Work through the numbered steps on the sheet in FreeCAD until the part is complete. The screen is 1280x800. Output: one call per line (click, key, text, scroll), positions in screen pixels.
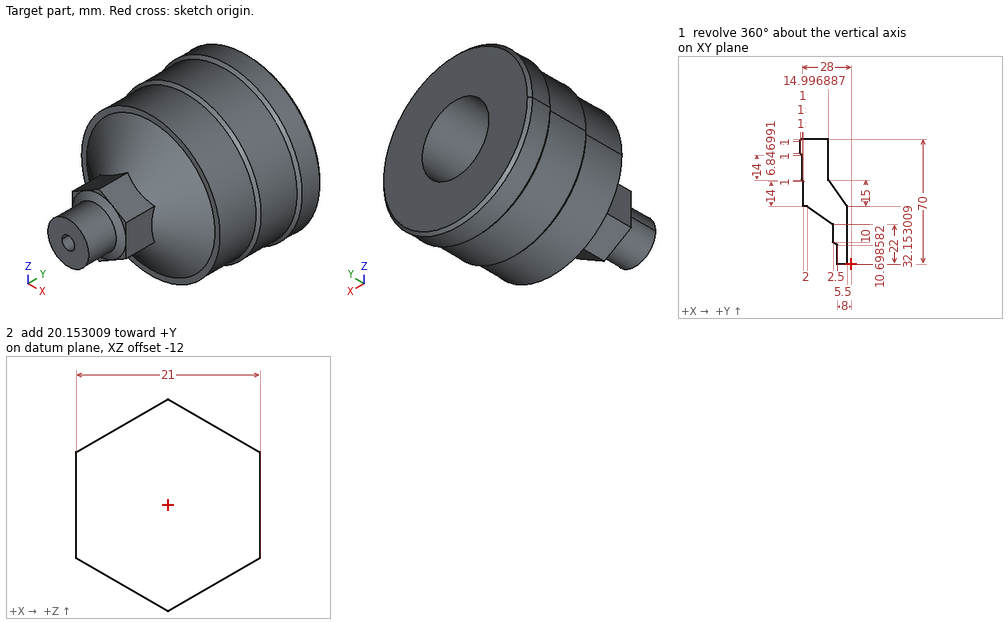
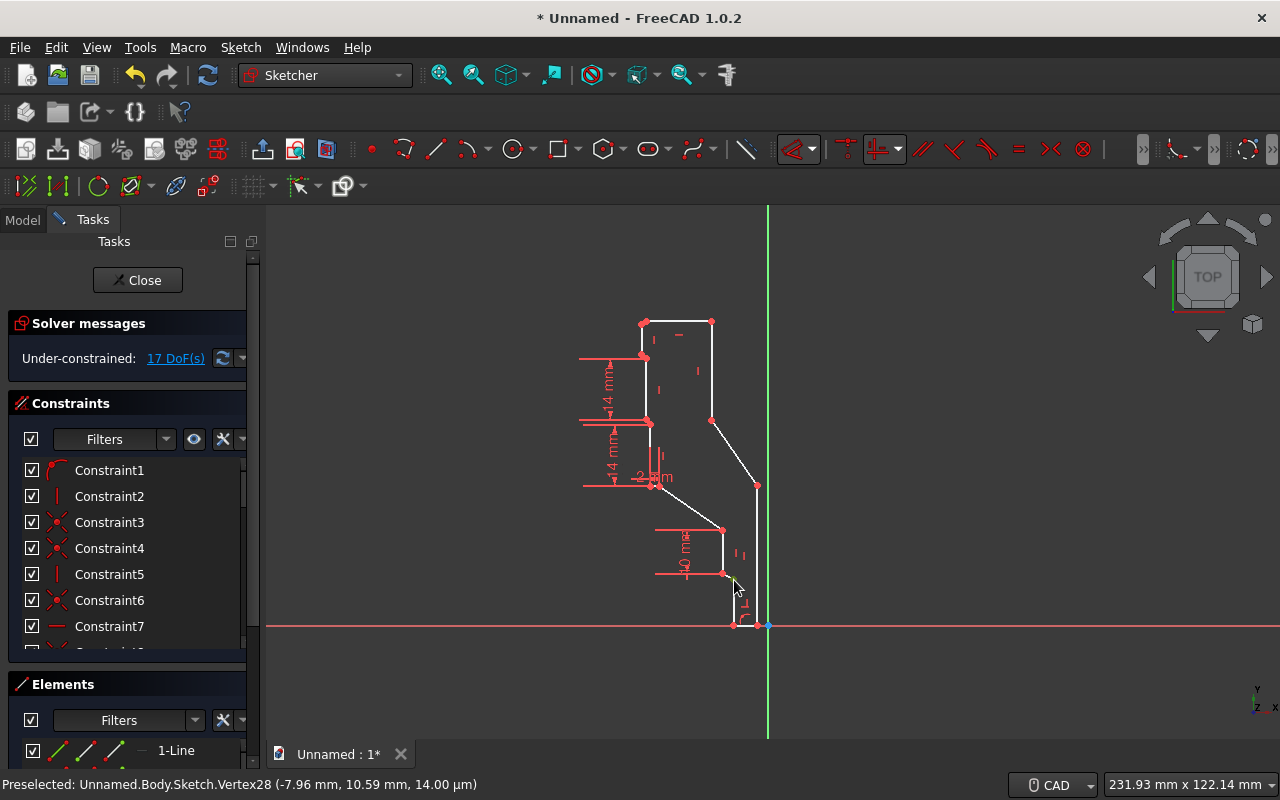
key(l)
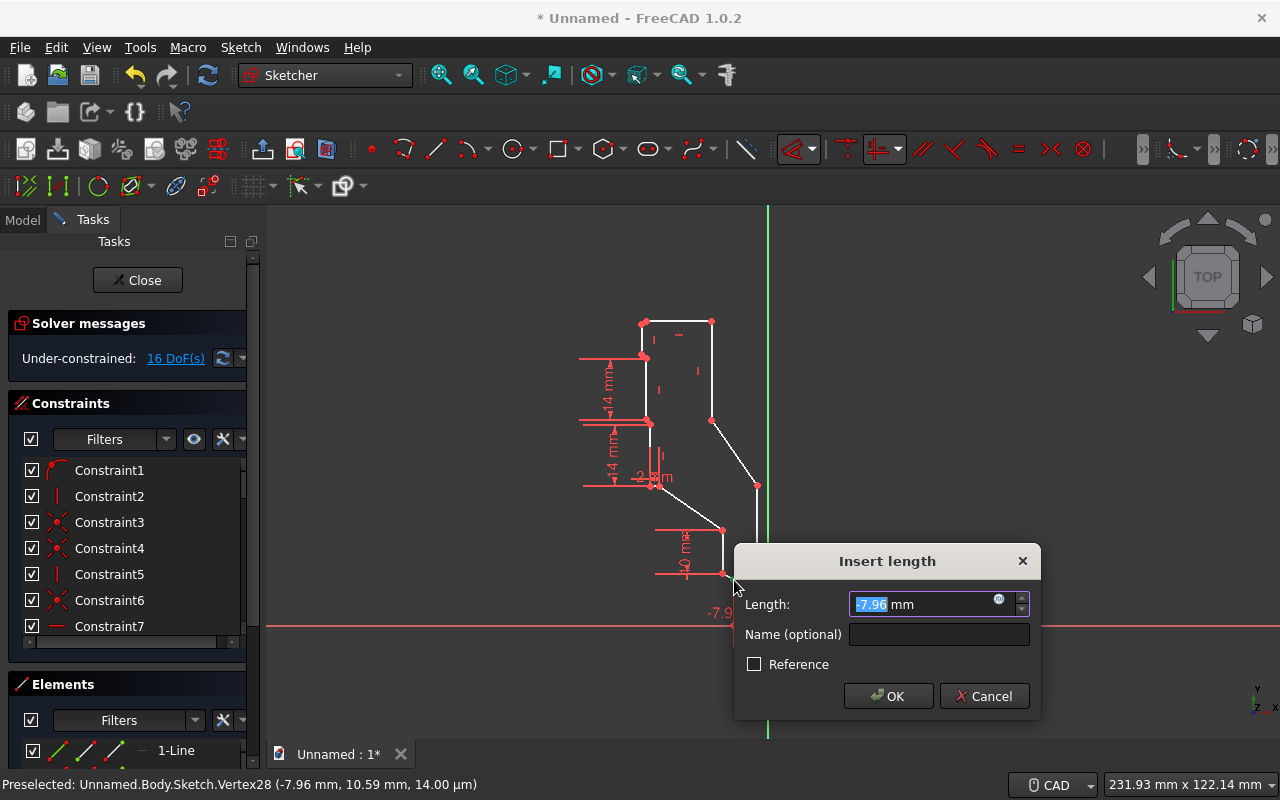
text(-8)
key(Return)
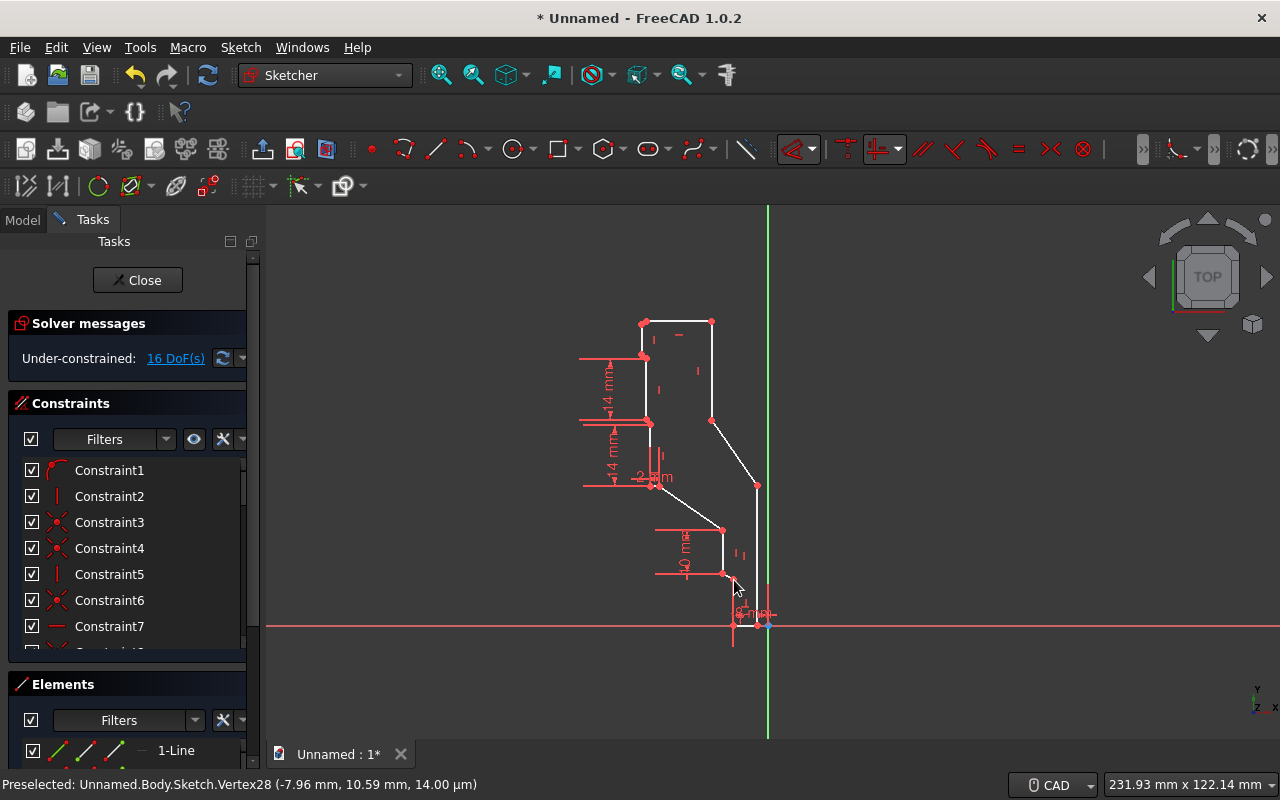
scroll(644, 323, up, 12)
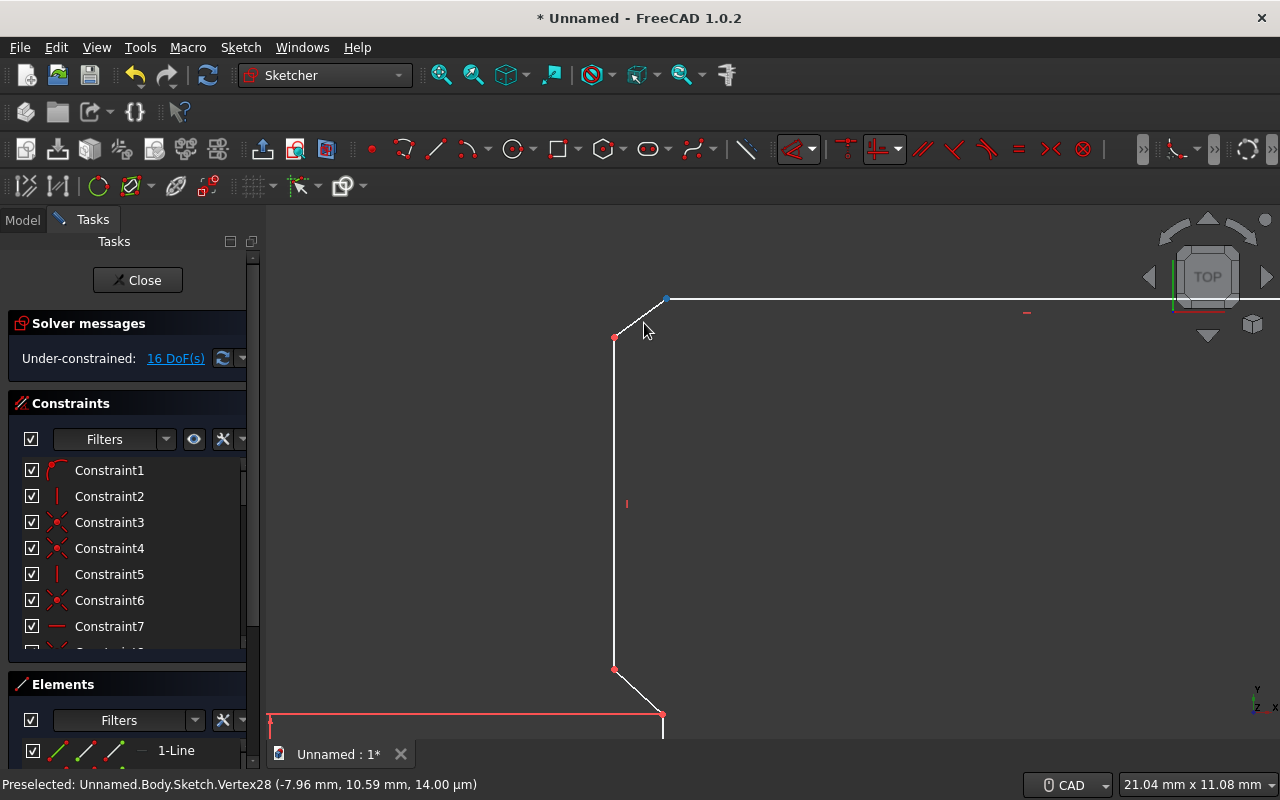
click(640, 318)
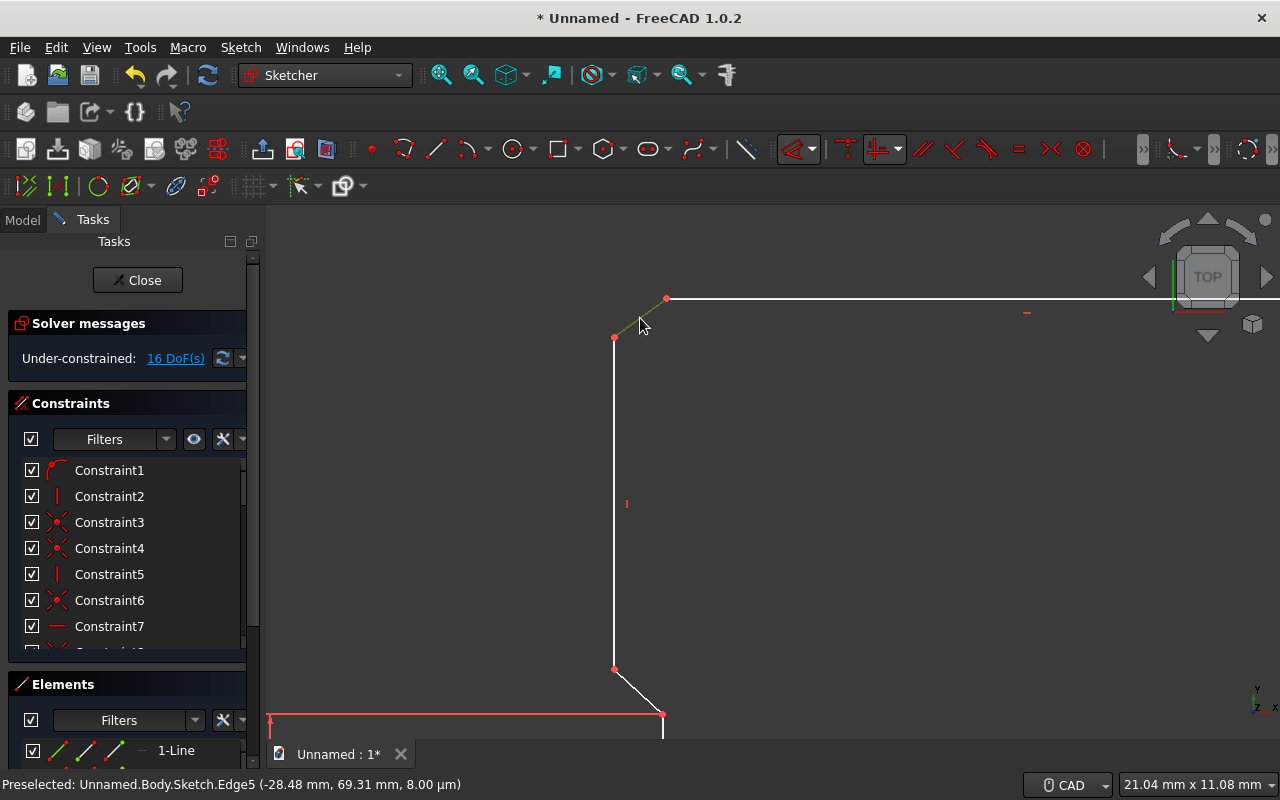
click(814, 150)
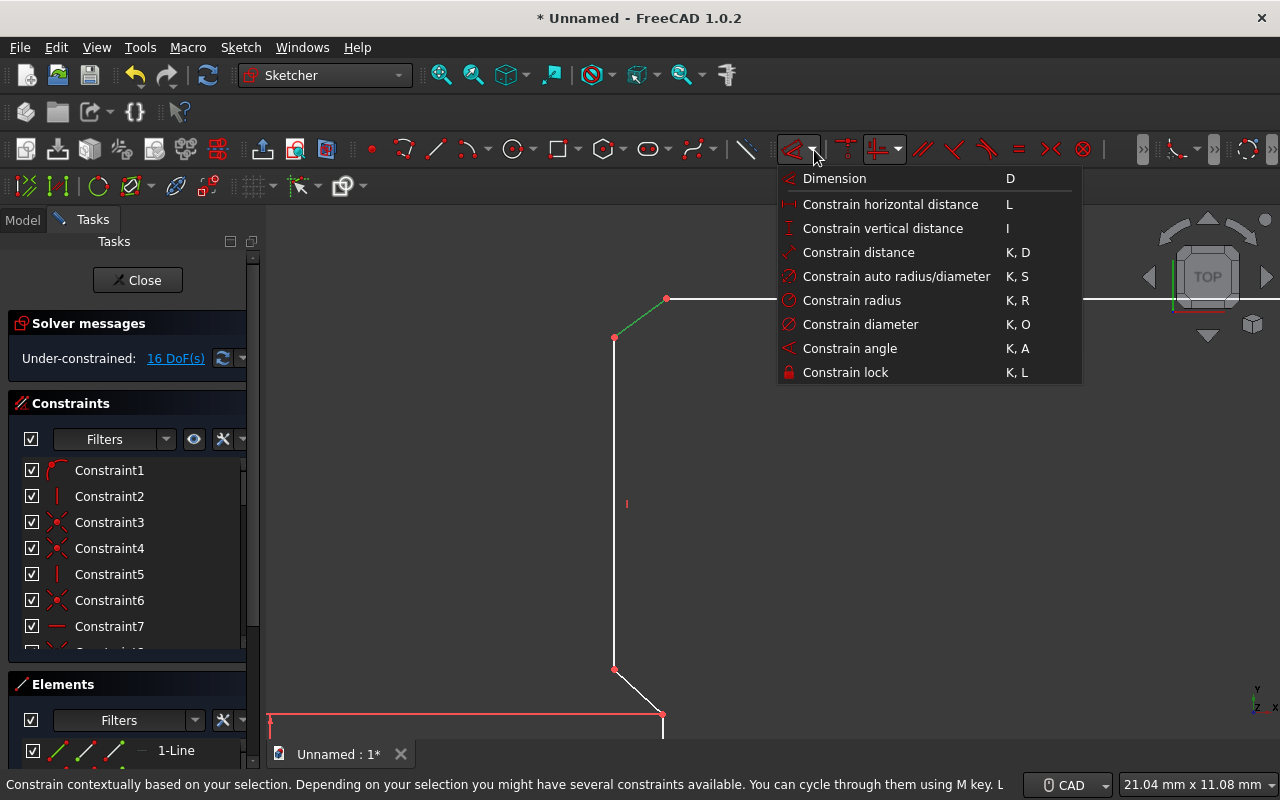
click(930, 204)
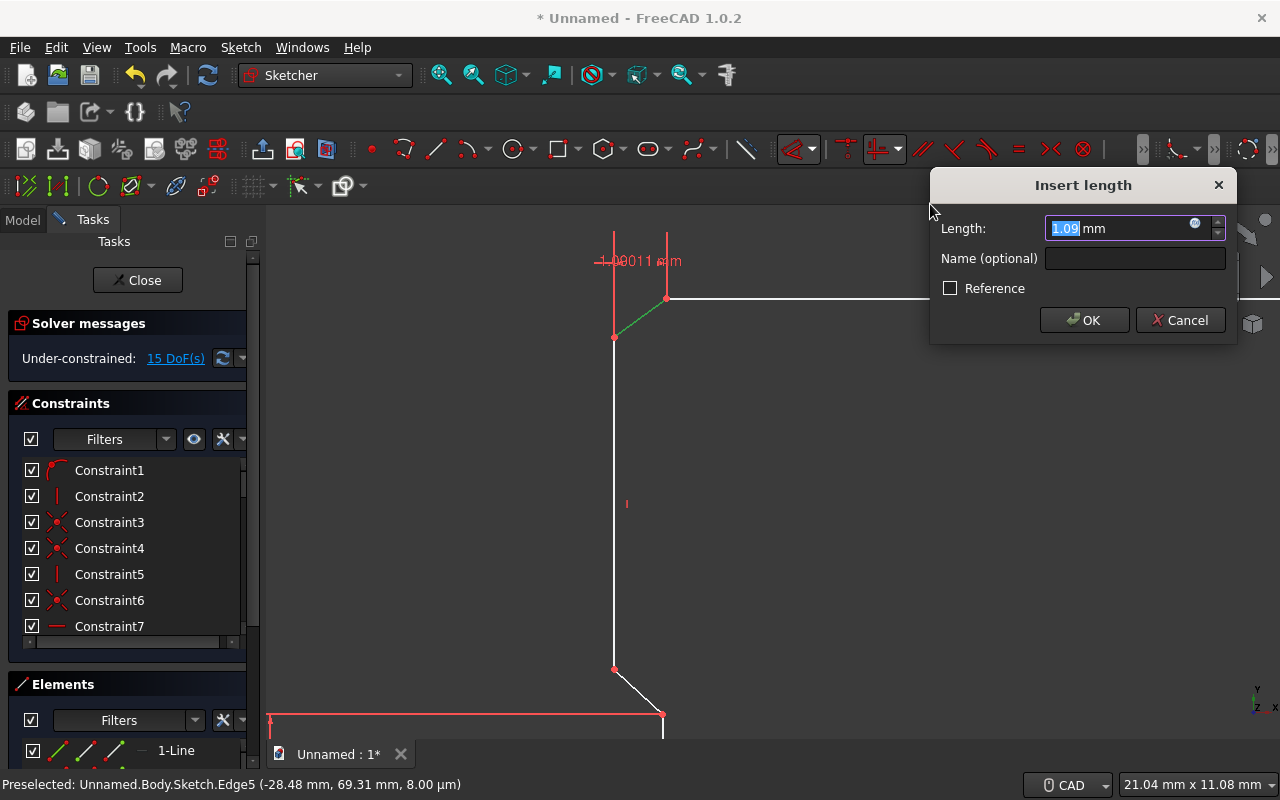
text(1)
key(Return)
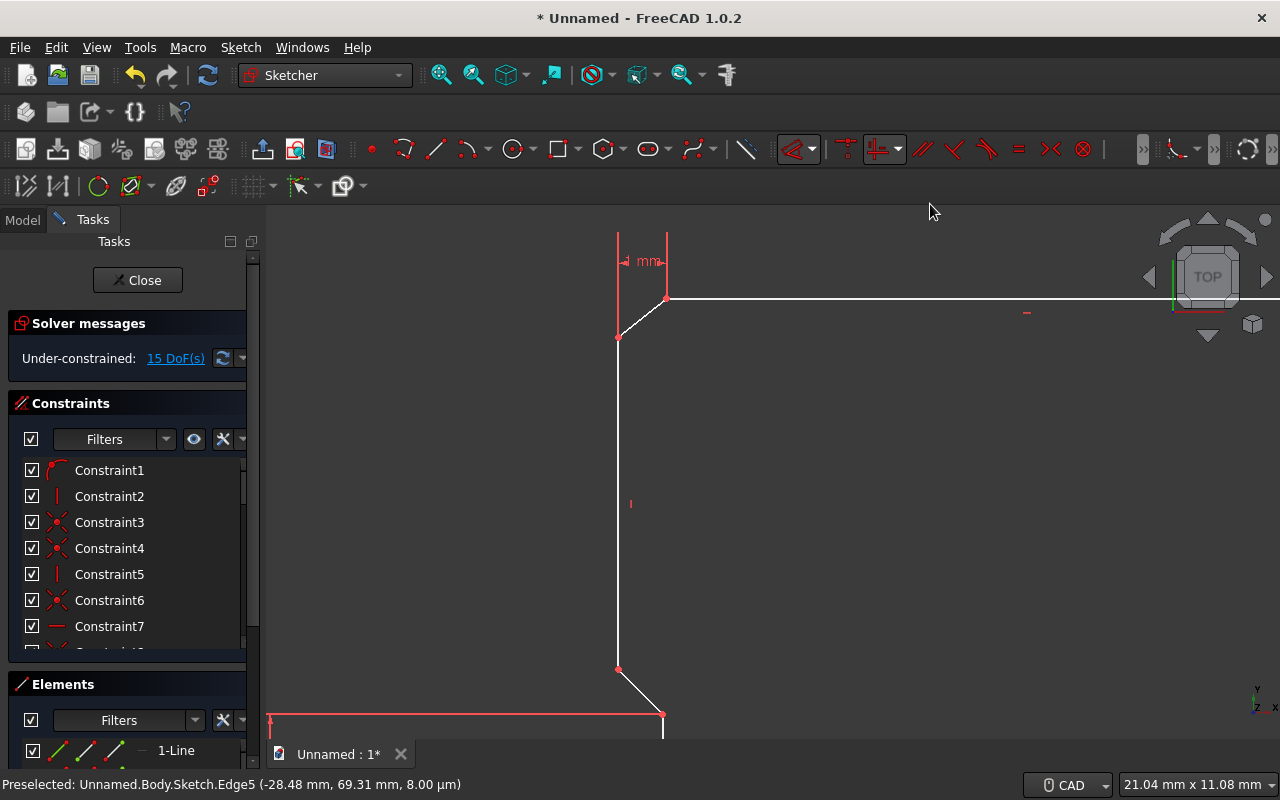
click(652, 310)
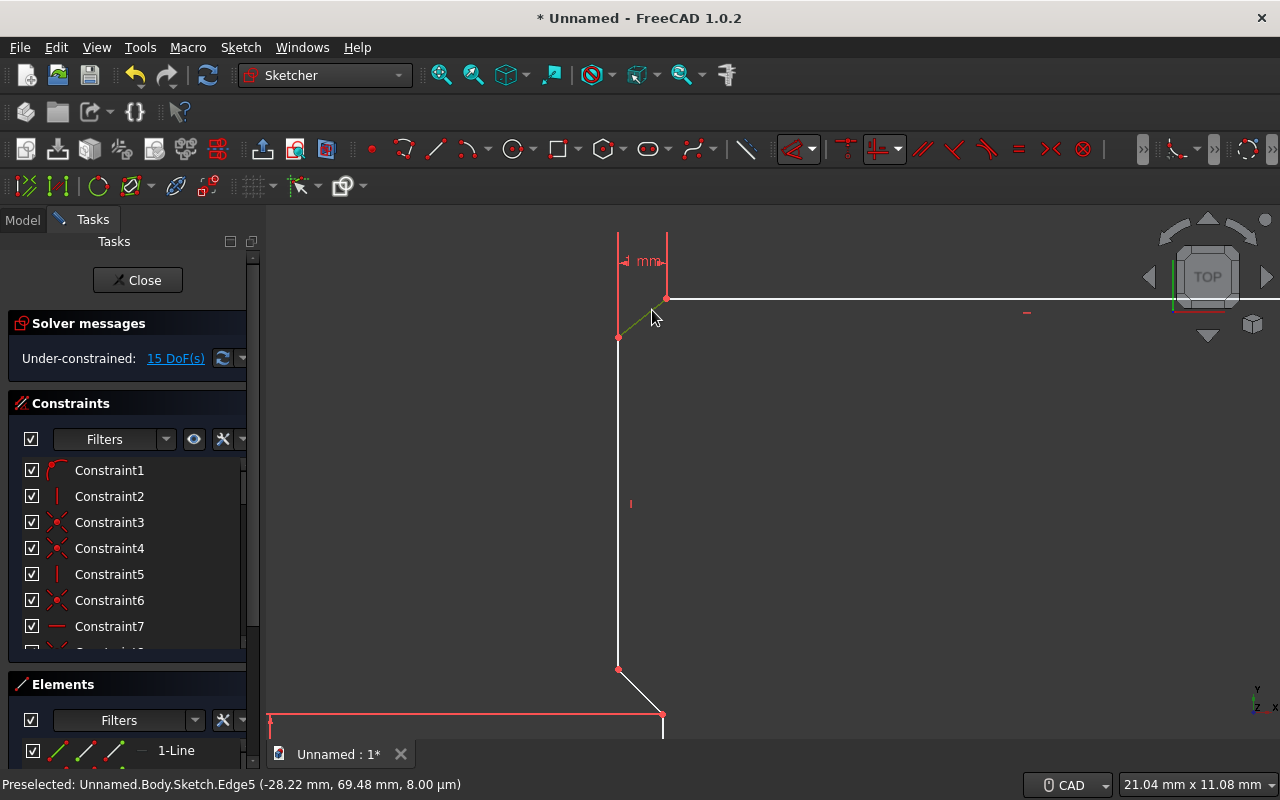
click(814, 150)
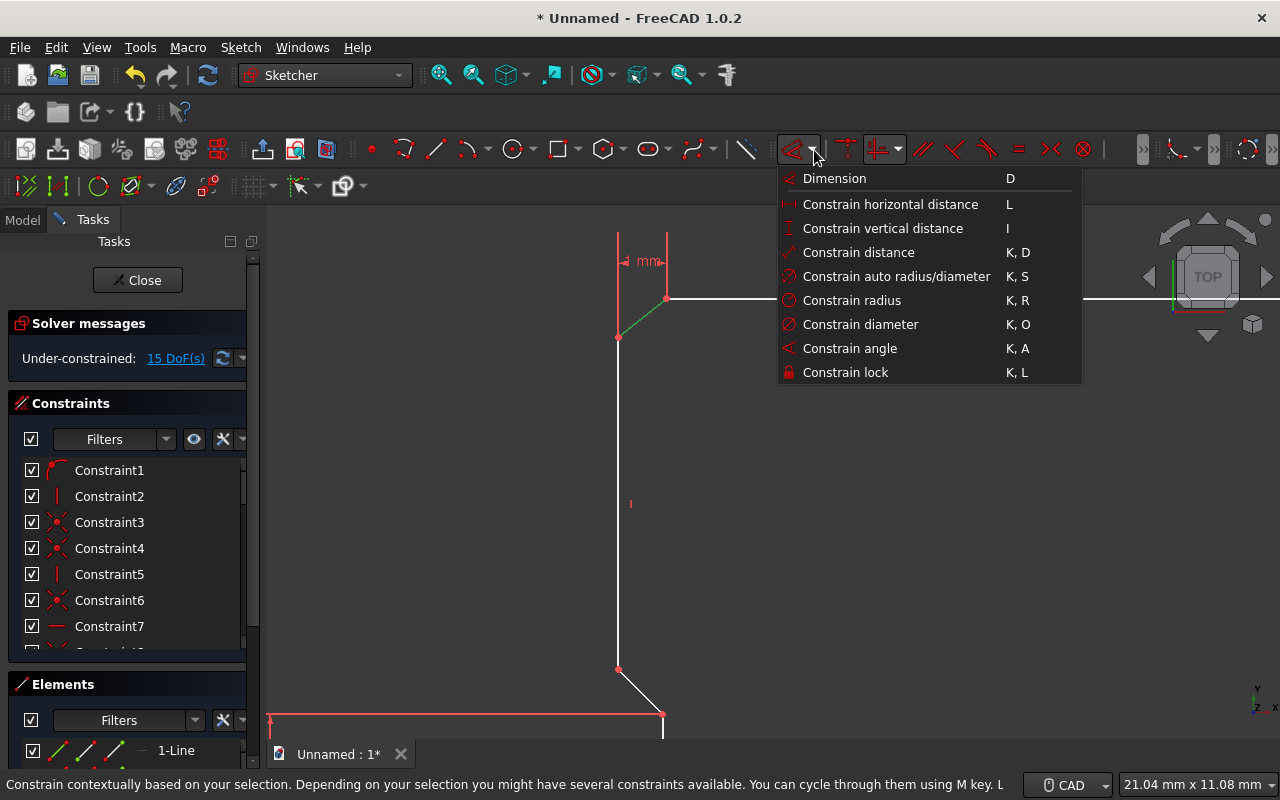
click(930, 228)